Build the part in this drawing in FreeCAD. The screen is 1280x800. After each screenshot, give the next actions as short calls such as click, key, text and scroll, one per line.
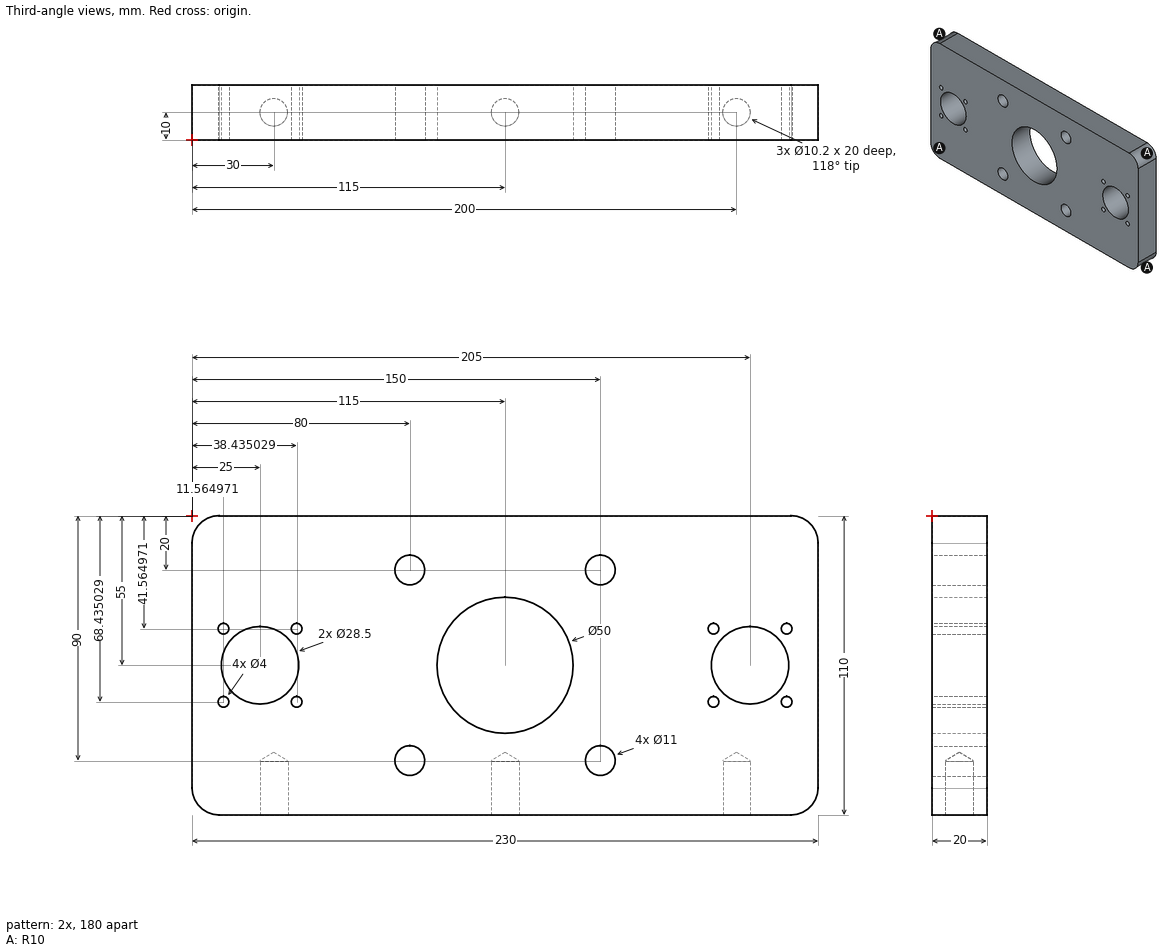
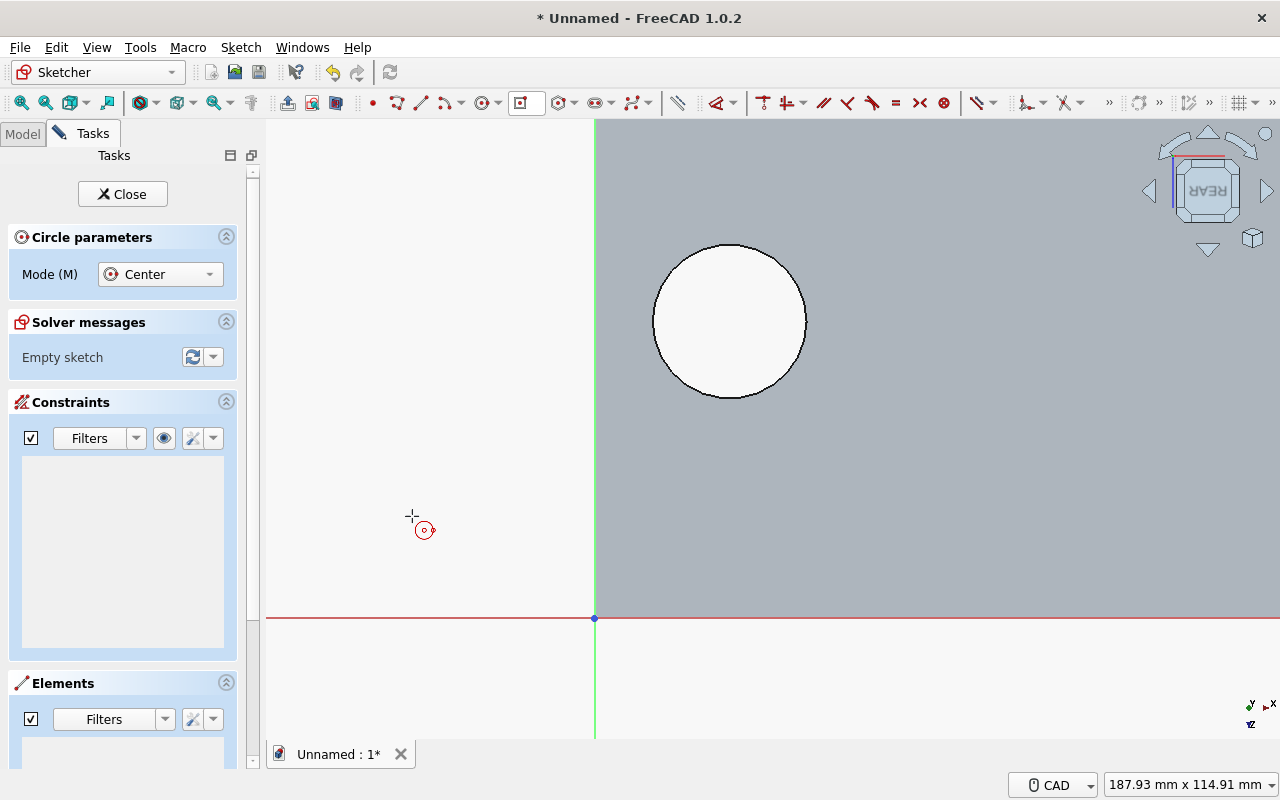
scroll(657, 249, up, 4)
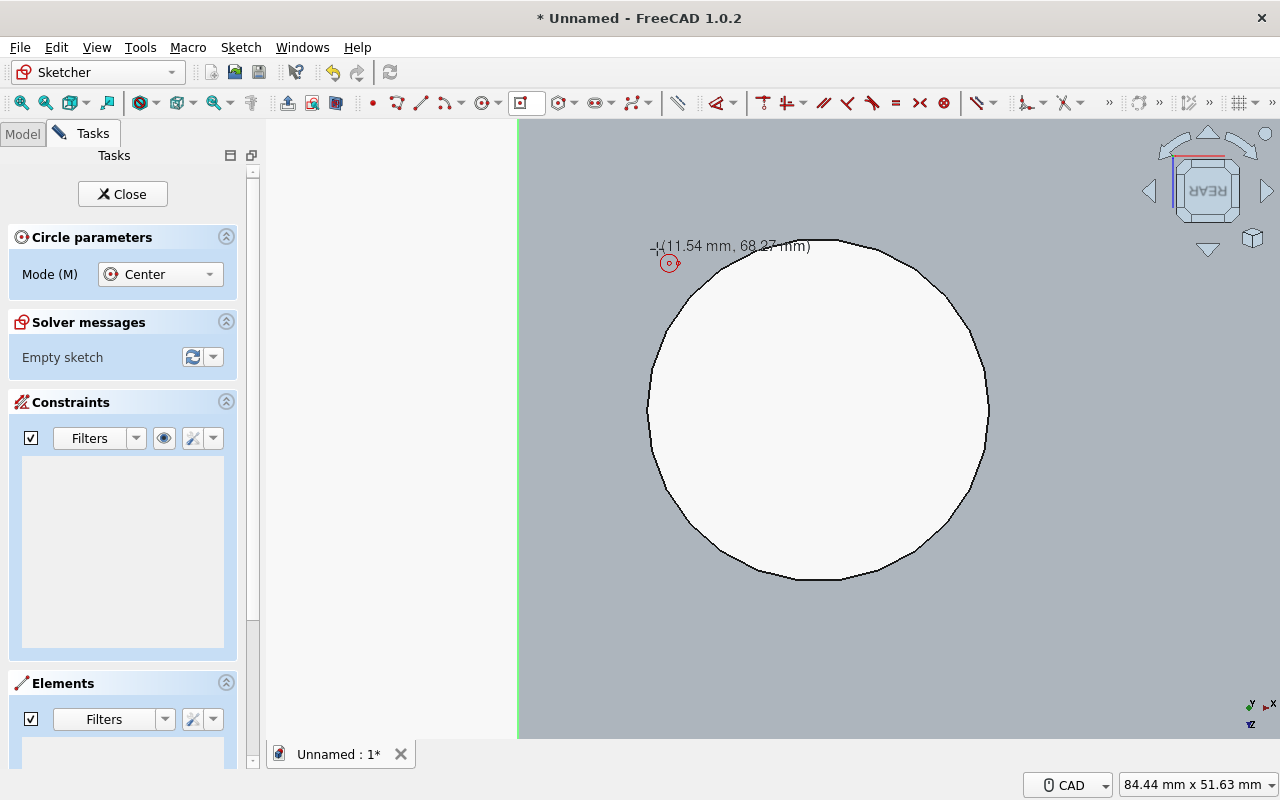
click(657, 249)
move(674, 232)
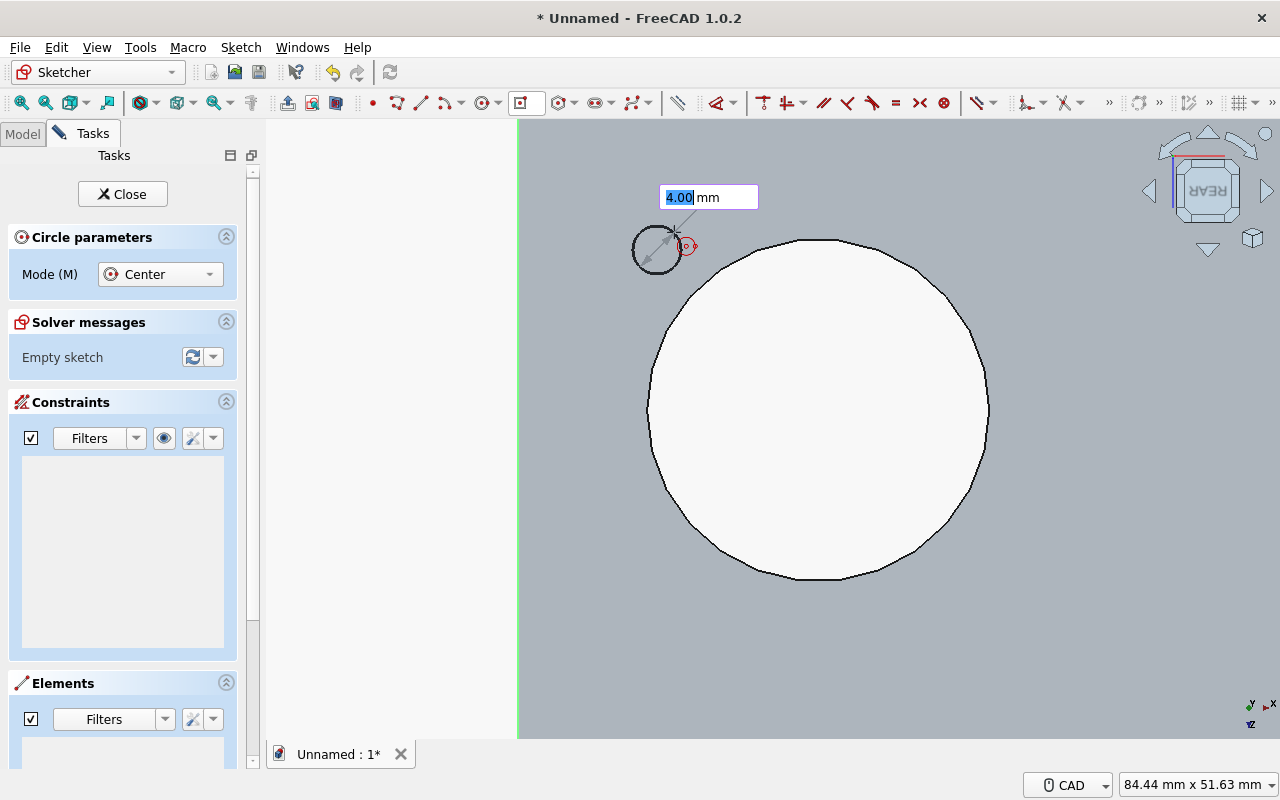
text(4)
key(Return)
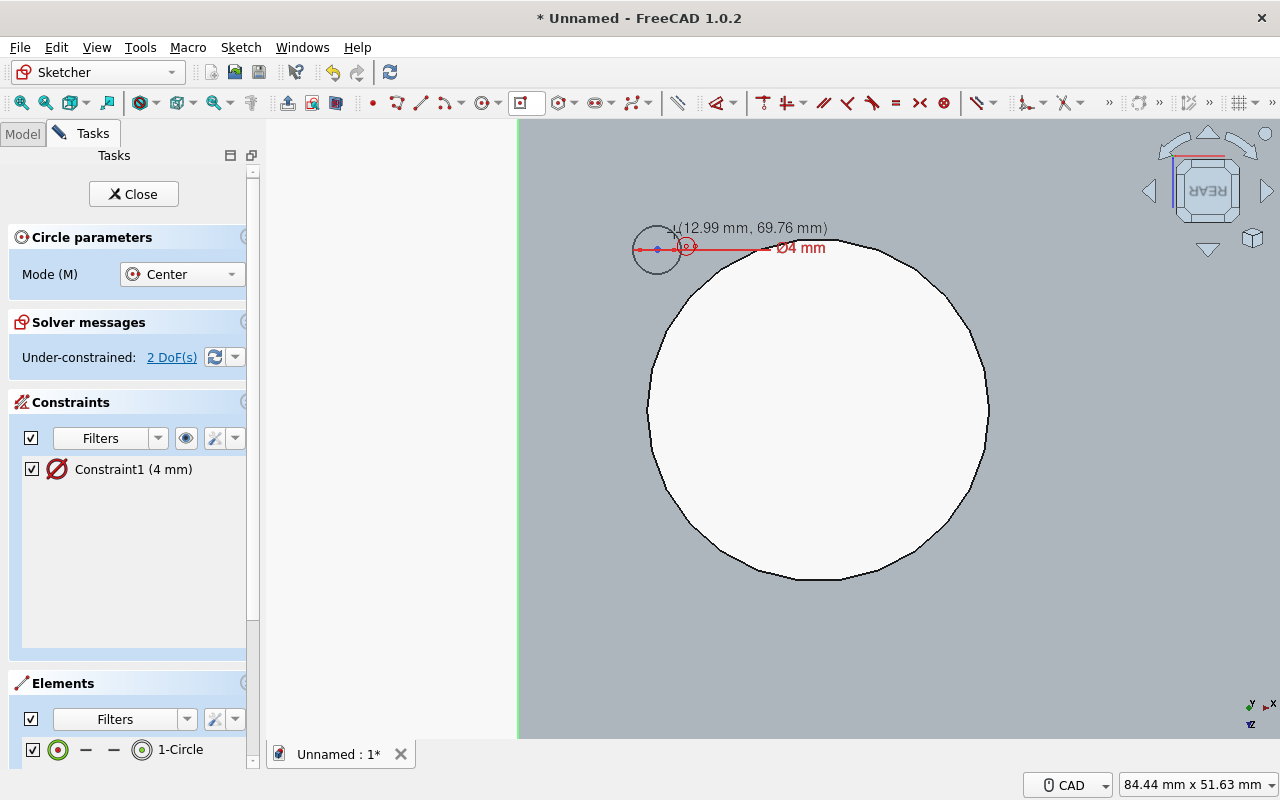
click(980, 249)
move(997, 232)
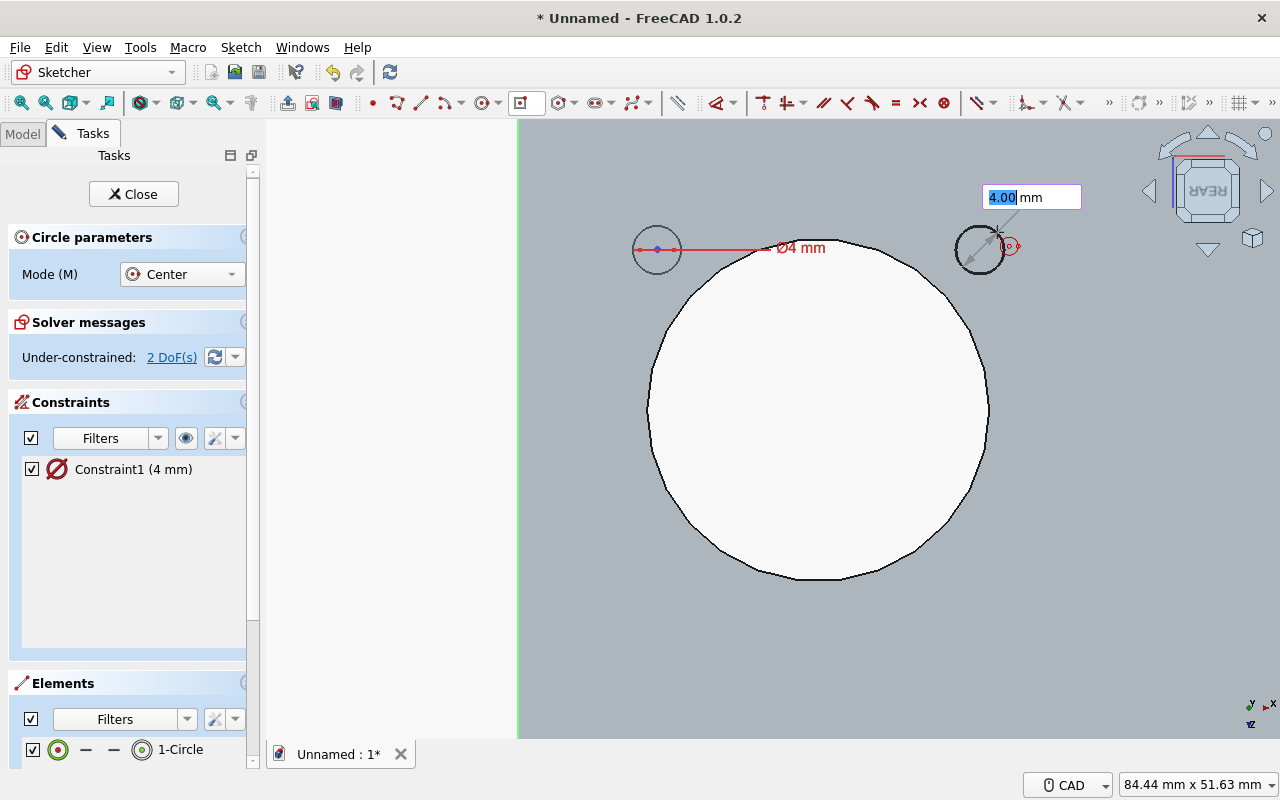
text(4)
key(Return)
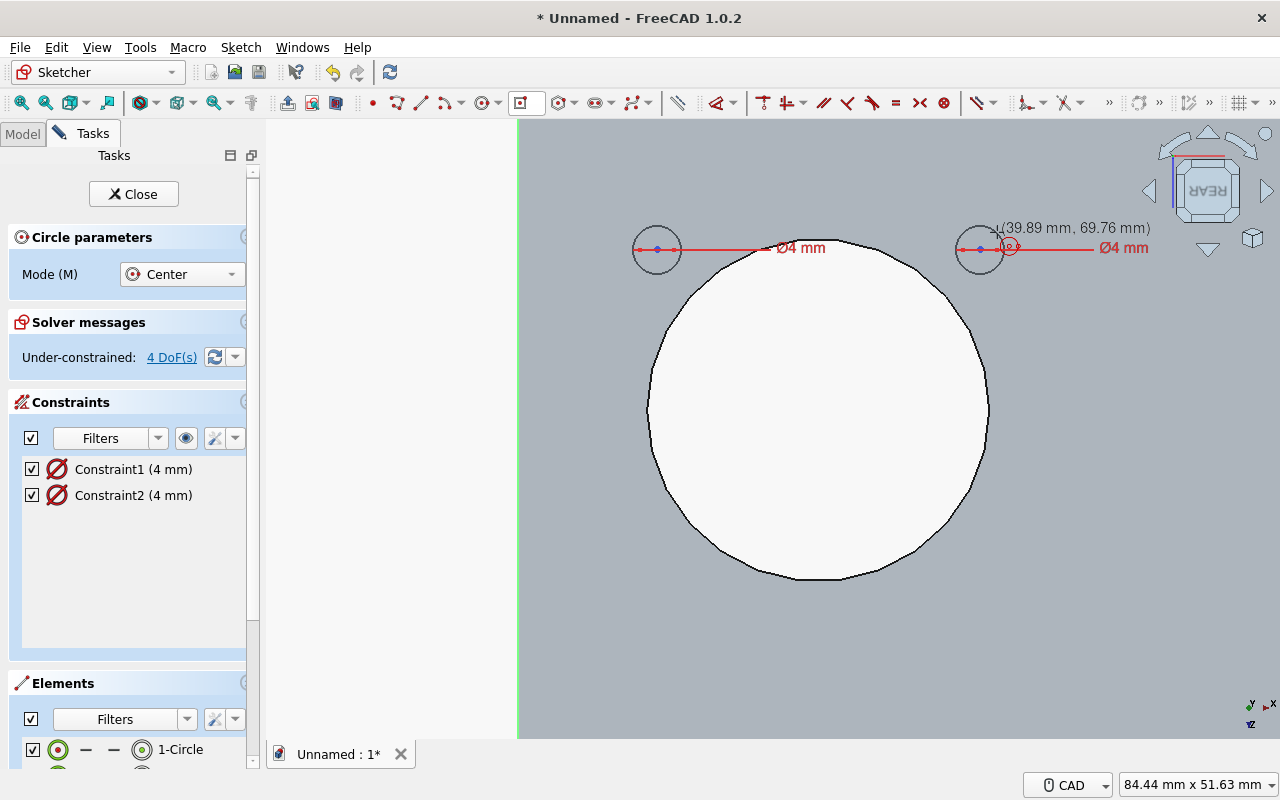
click(980, 572)
move(997, 555)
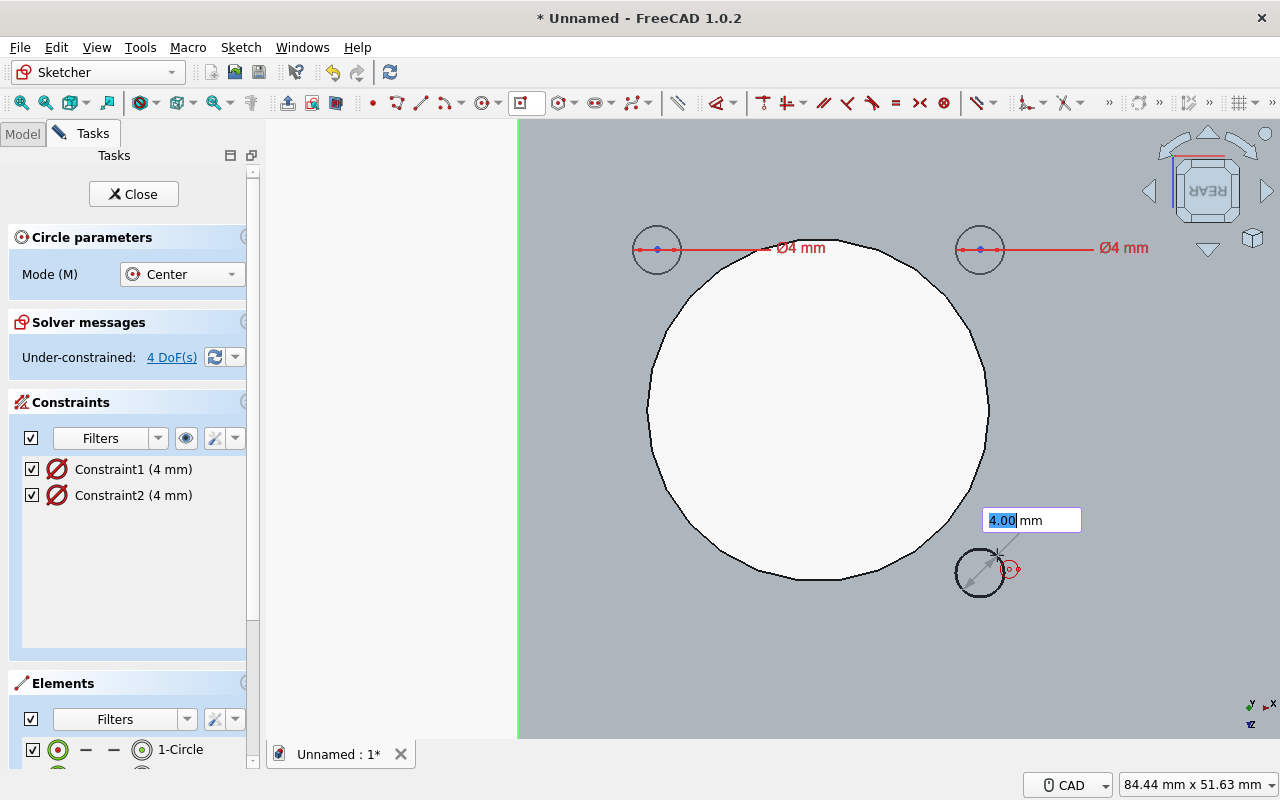
text(4)
key(Return)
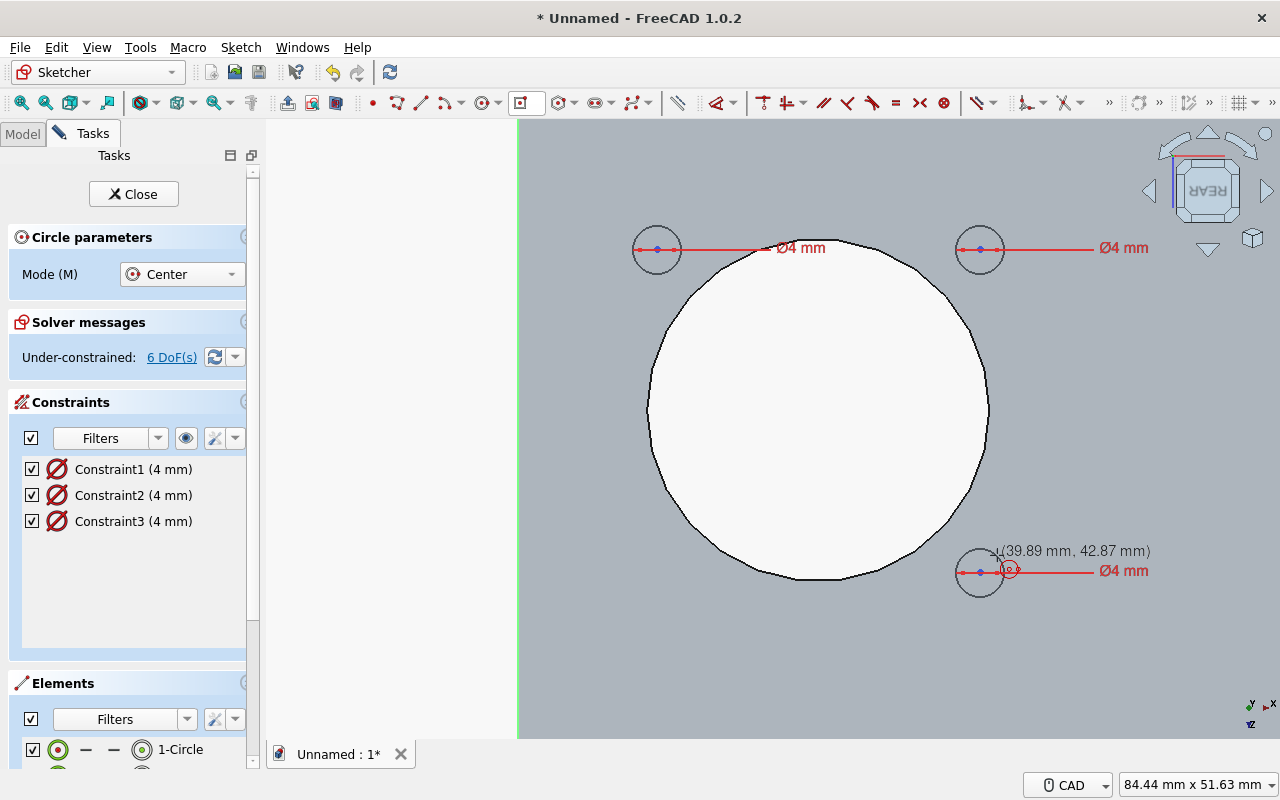
click(657, 572)
move(674, 555)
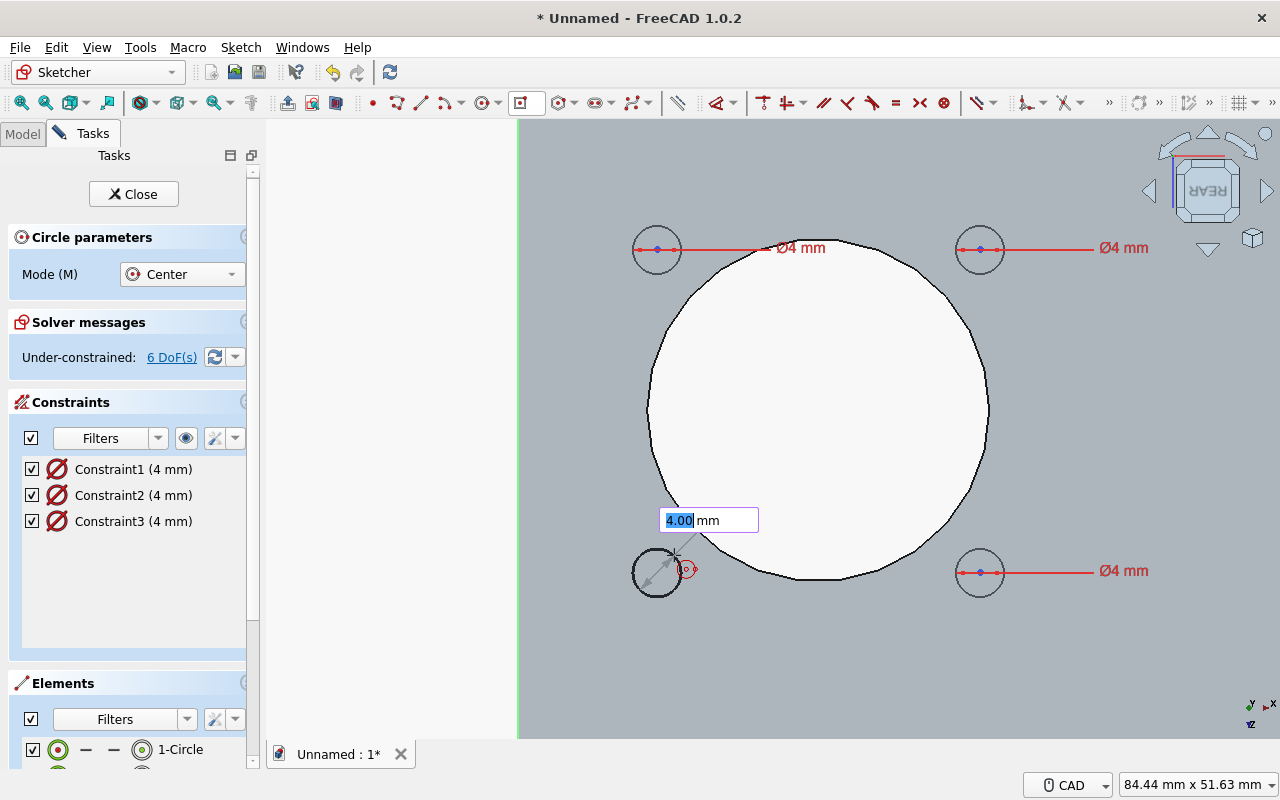
text(4)
key(Return)
key(Escape)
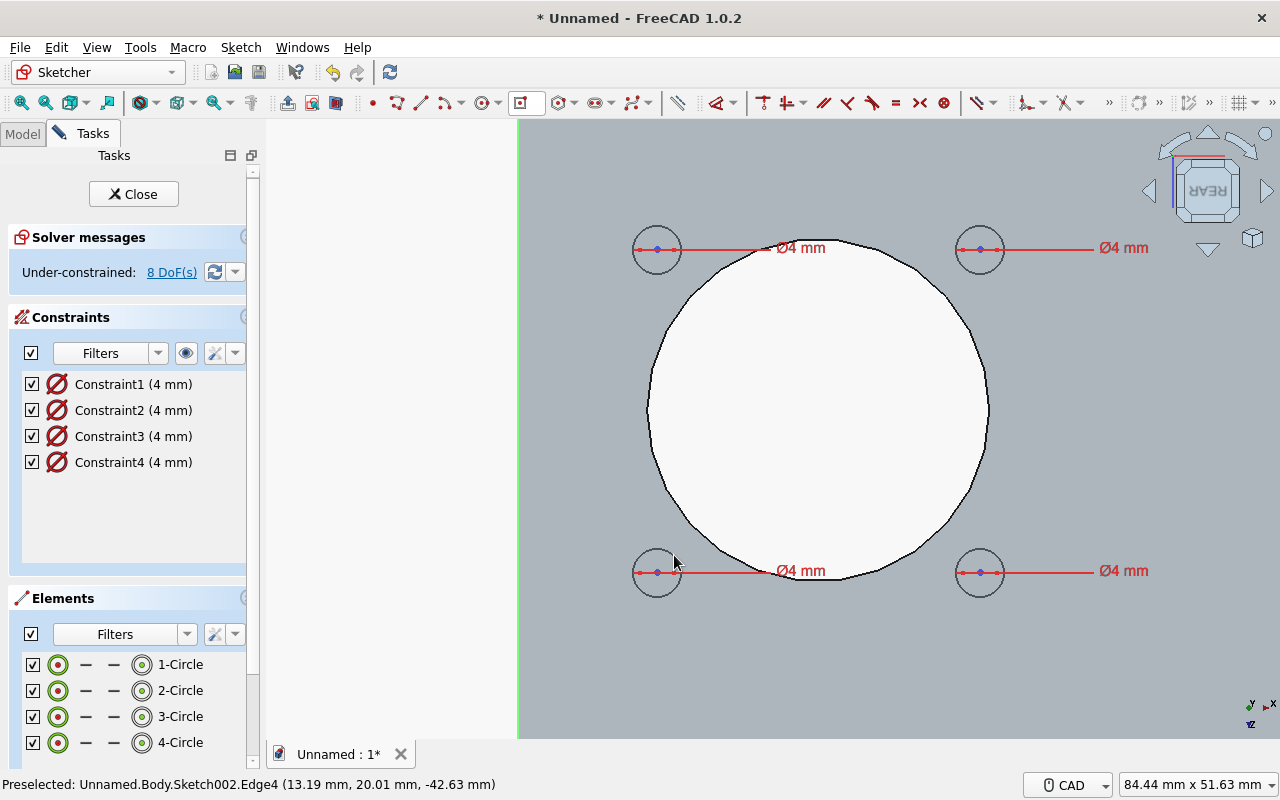
key(d)